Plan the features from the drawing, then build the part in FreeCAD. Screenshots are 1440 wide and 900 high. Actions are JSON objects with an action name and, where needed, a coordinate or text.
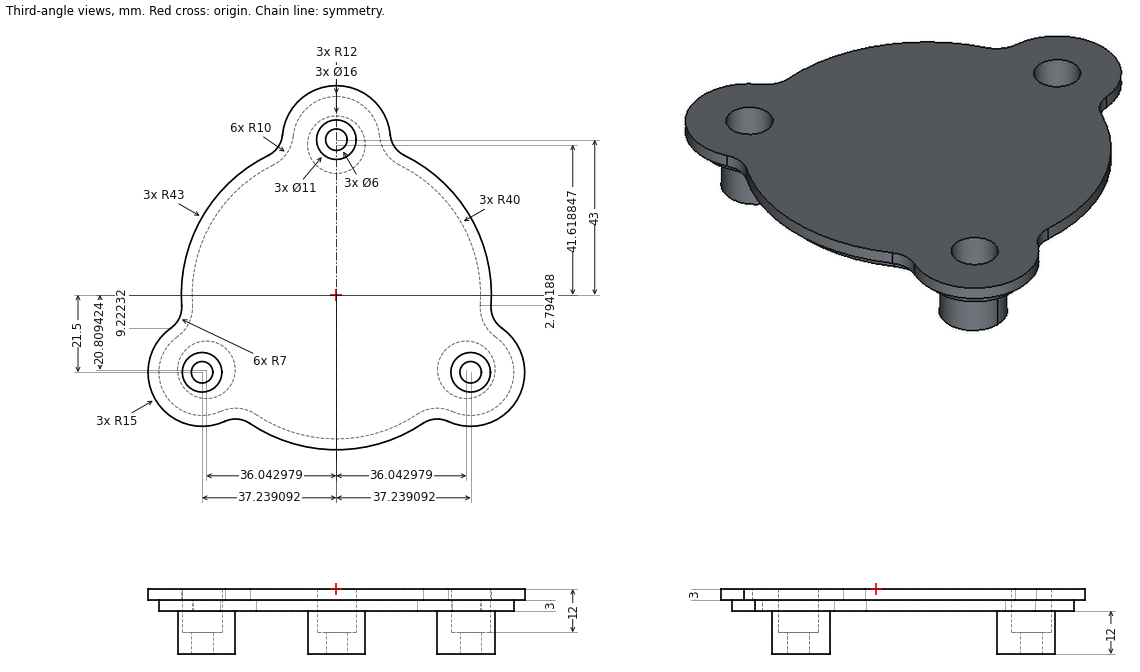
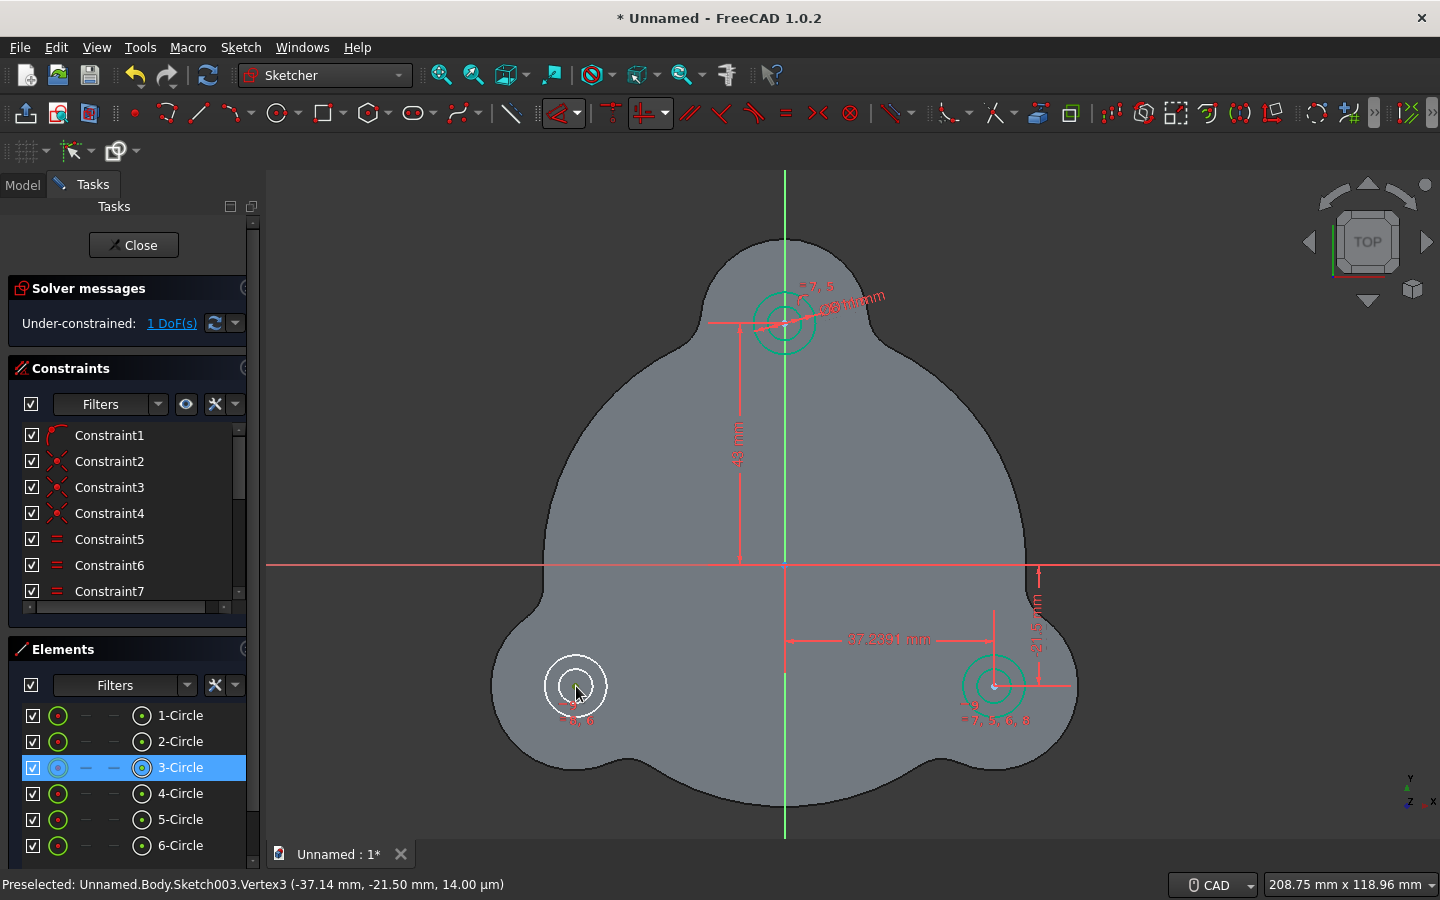
{"action": "left_click", "coordinate": [580, 114]}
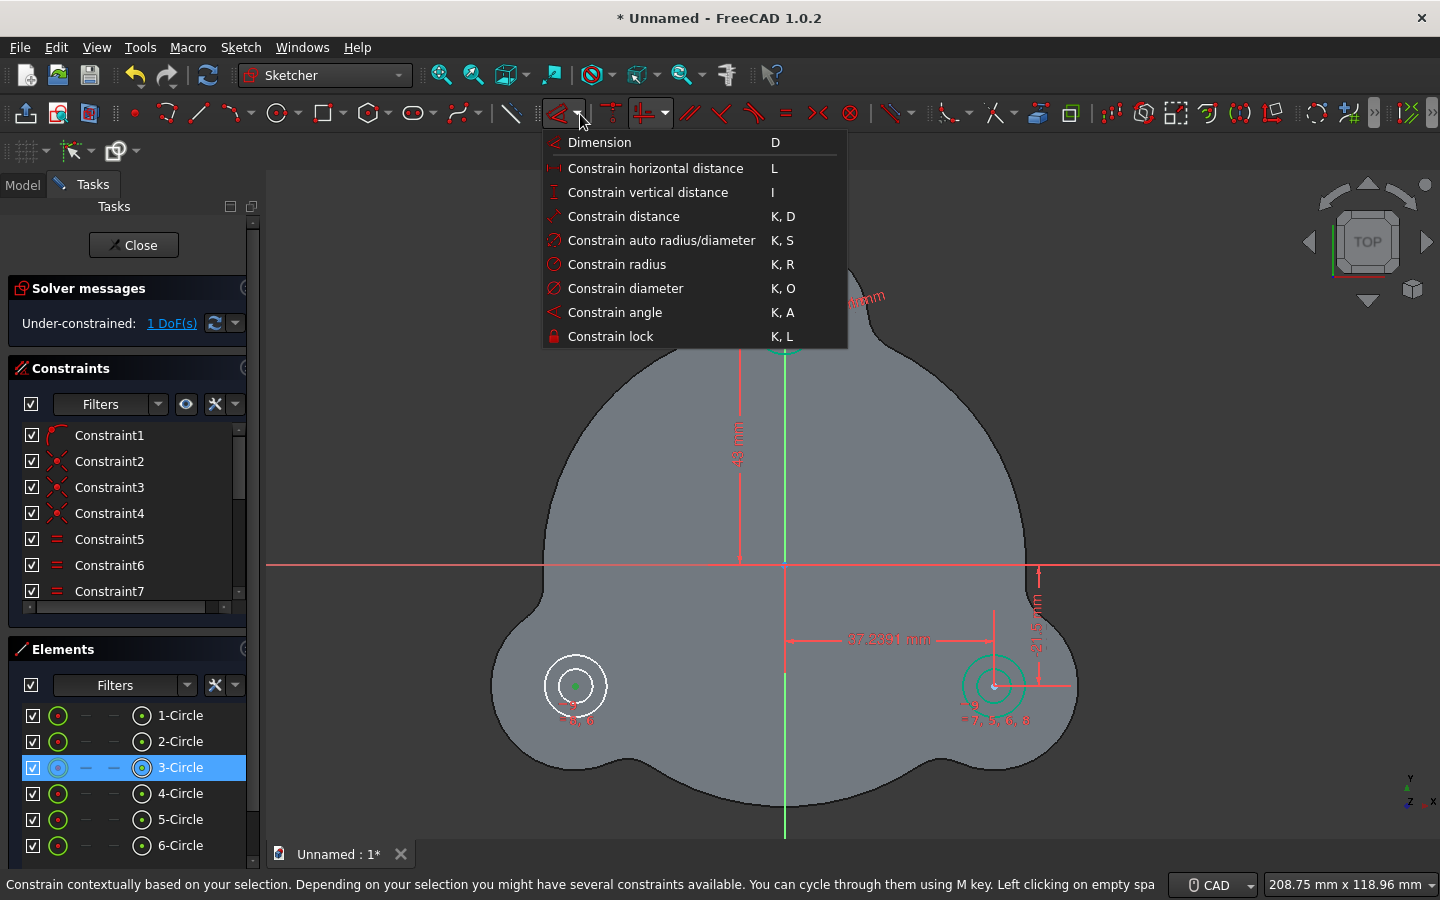
{"action": "left_click", "coordinate": [695, 168]}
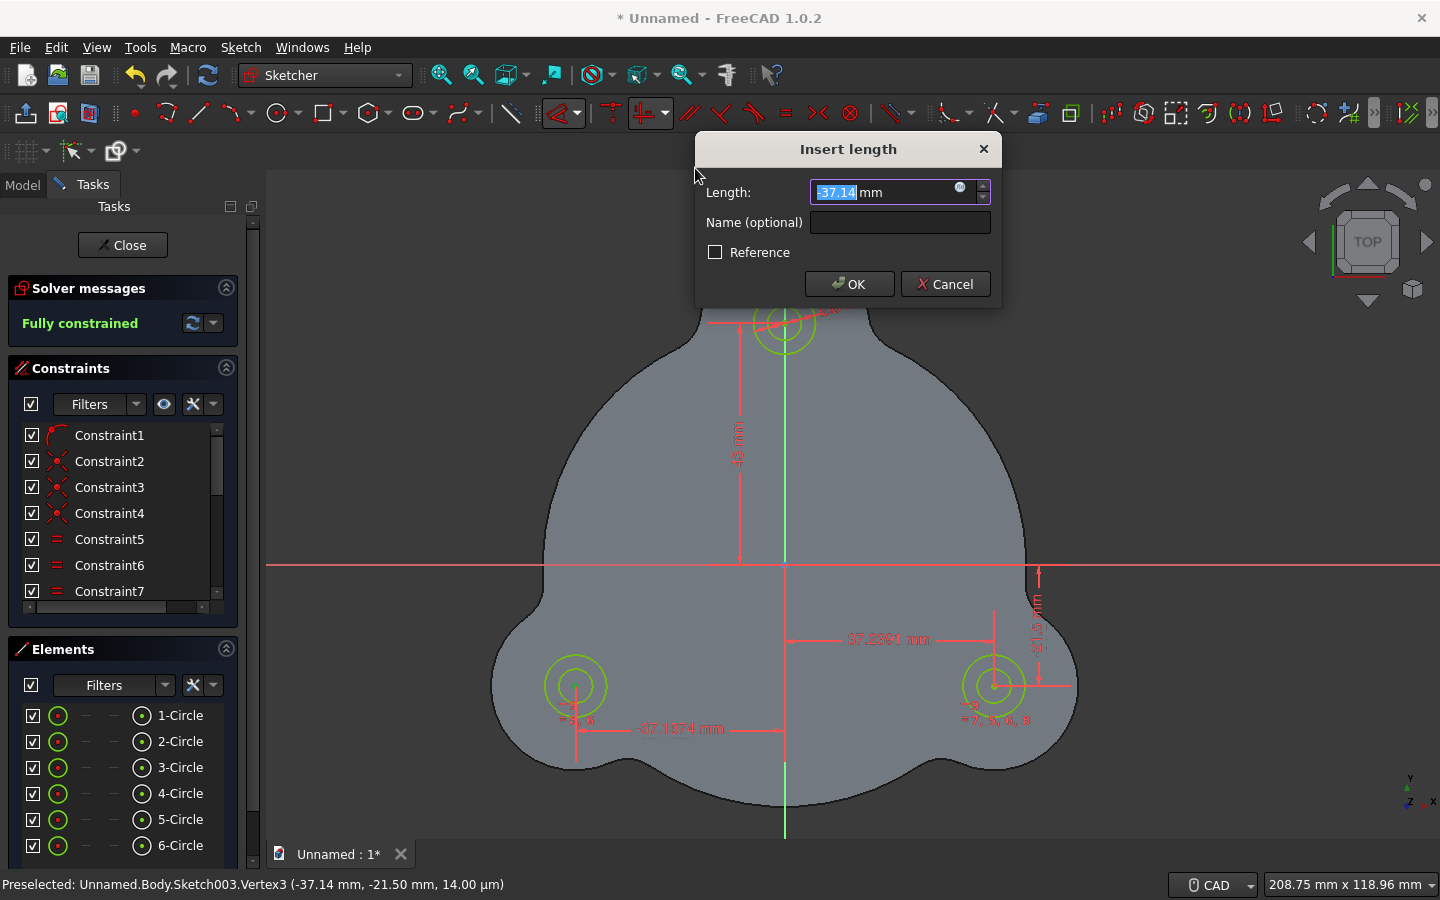
{"action": "type", "text": "-37.239092"}
{"action": "key", "text": "Return"}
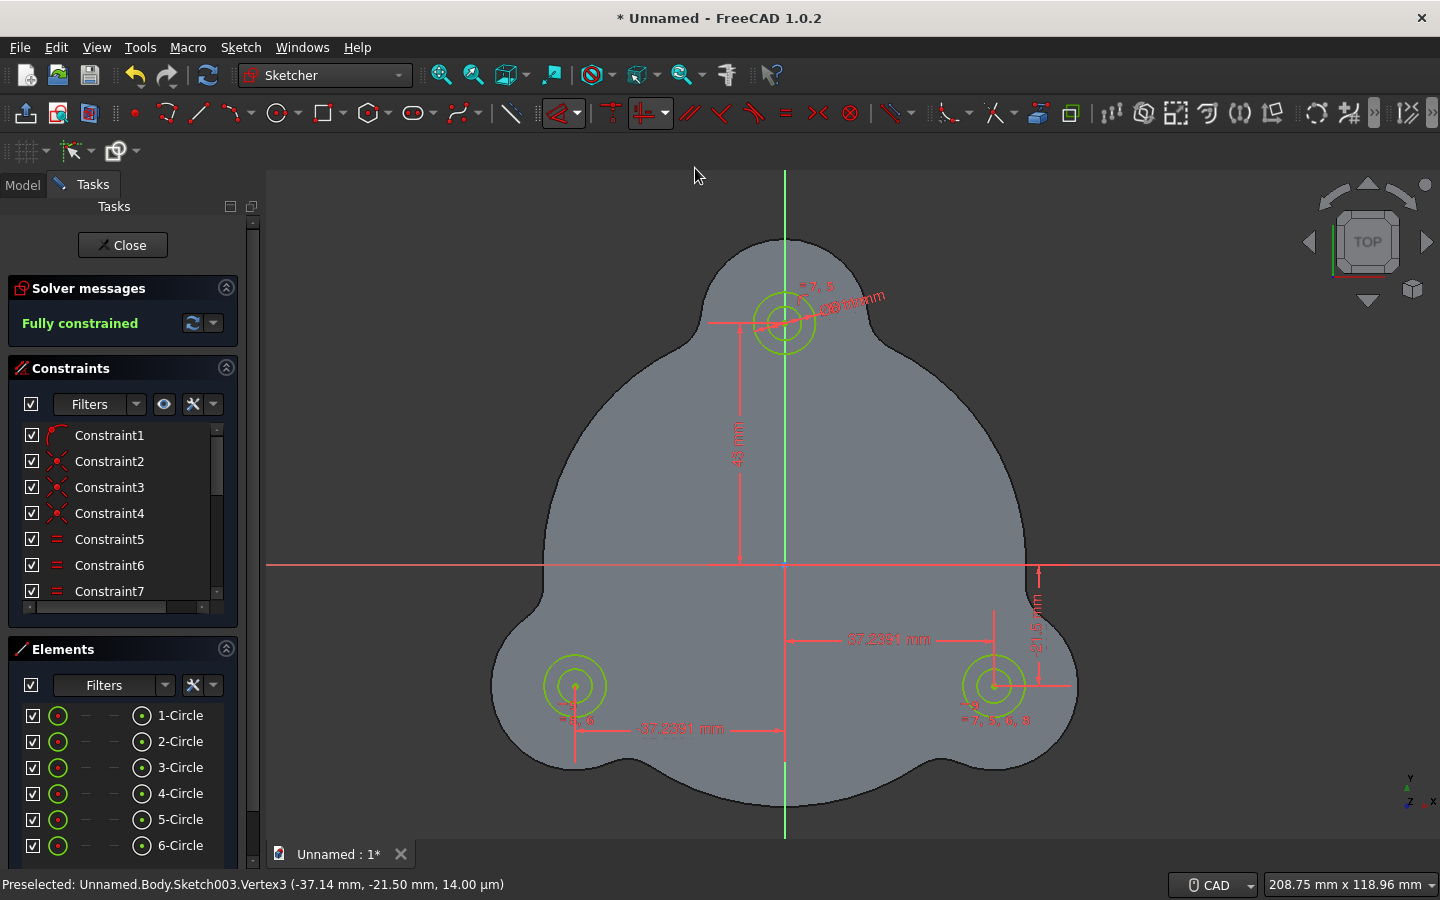
{"action": "left_click", "coordinate": [123, 245]}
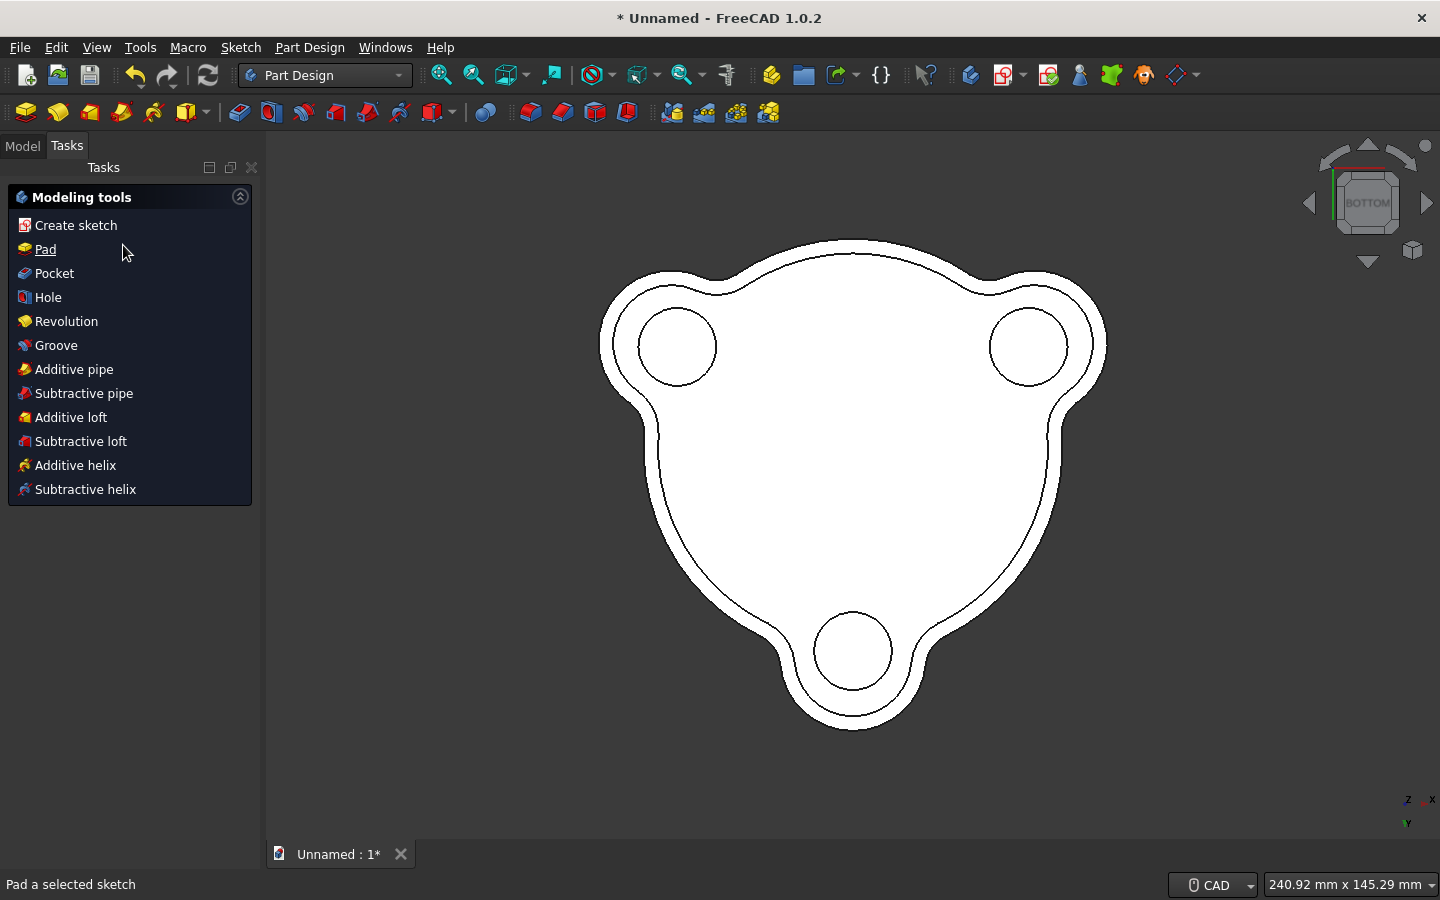
{"action": "left_click", "coordinate": [240, 112]}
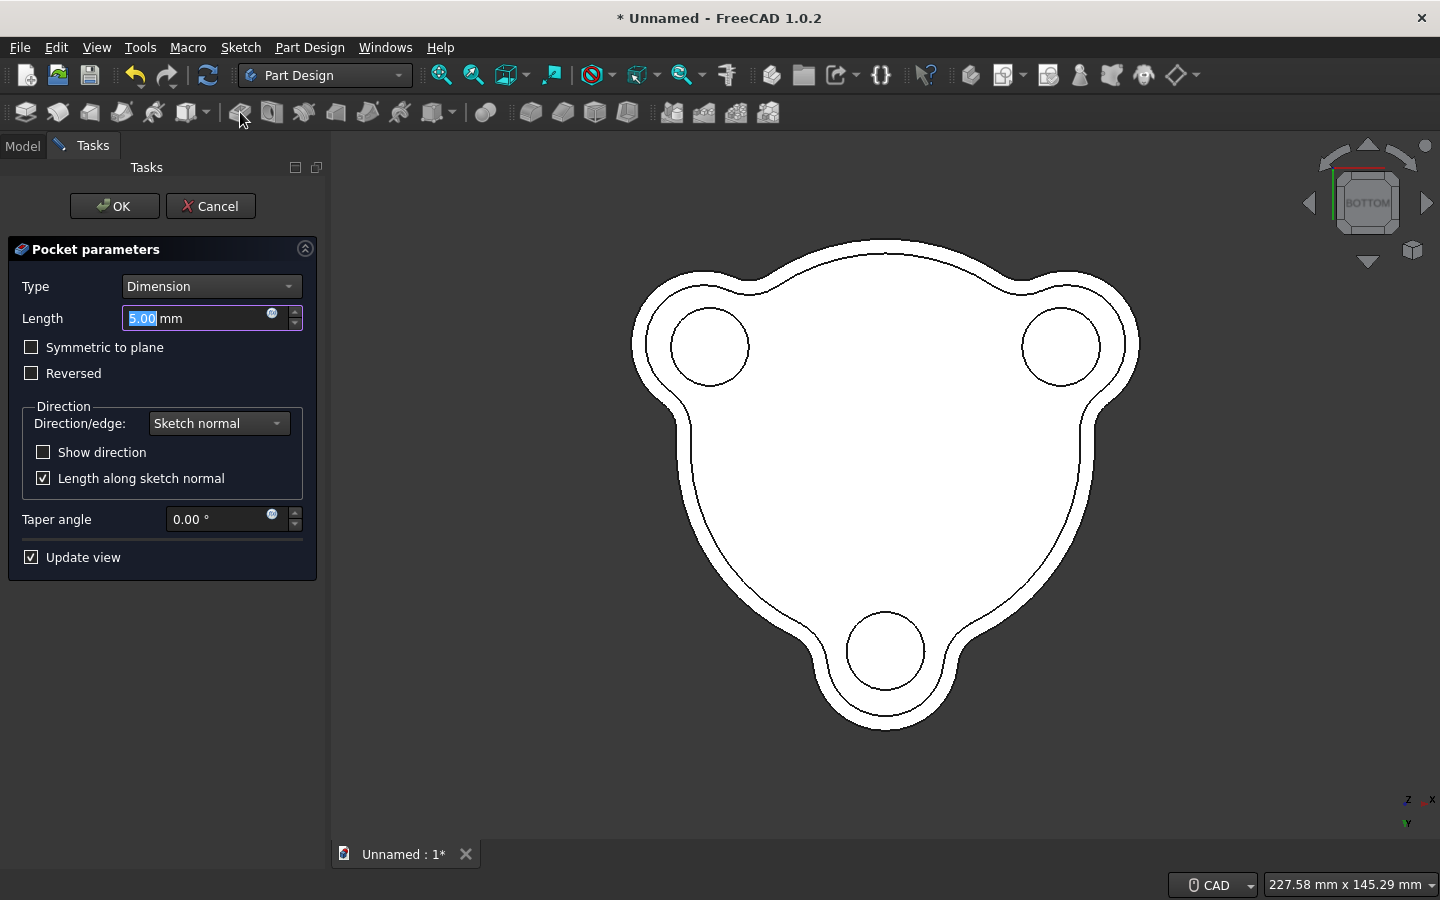
{"action": "type", "text": "12"}
{"action": "key", "text": "Tab"}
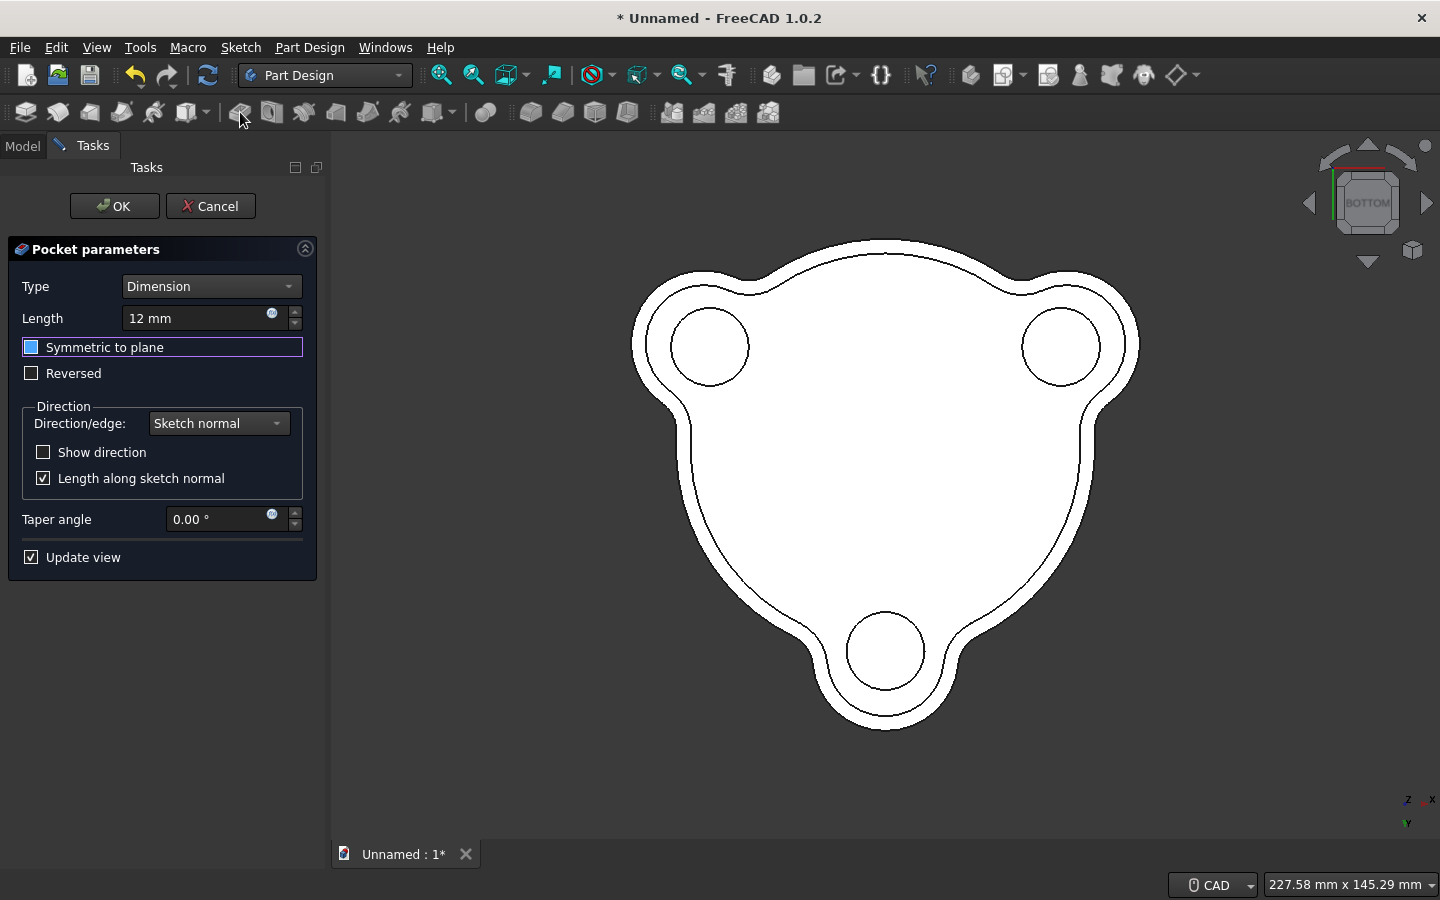
{"action": "left_click", "coordinate": [115, 206]}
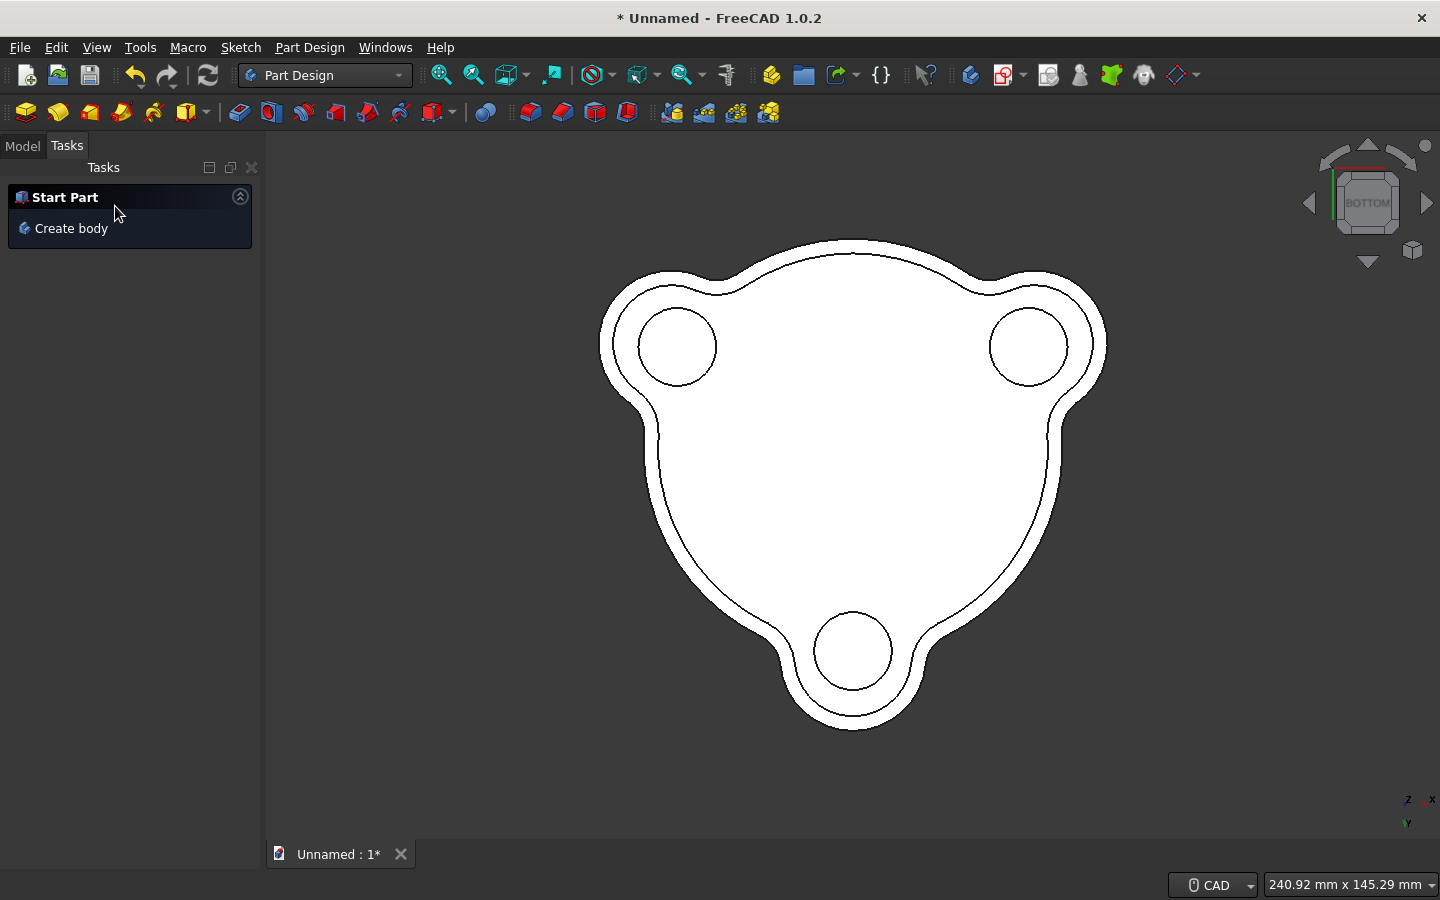
{"action": "left_click", "coordinate": [1004, 76]}